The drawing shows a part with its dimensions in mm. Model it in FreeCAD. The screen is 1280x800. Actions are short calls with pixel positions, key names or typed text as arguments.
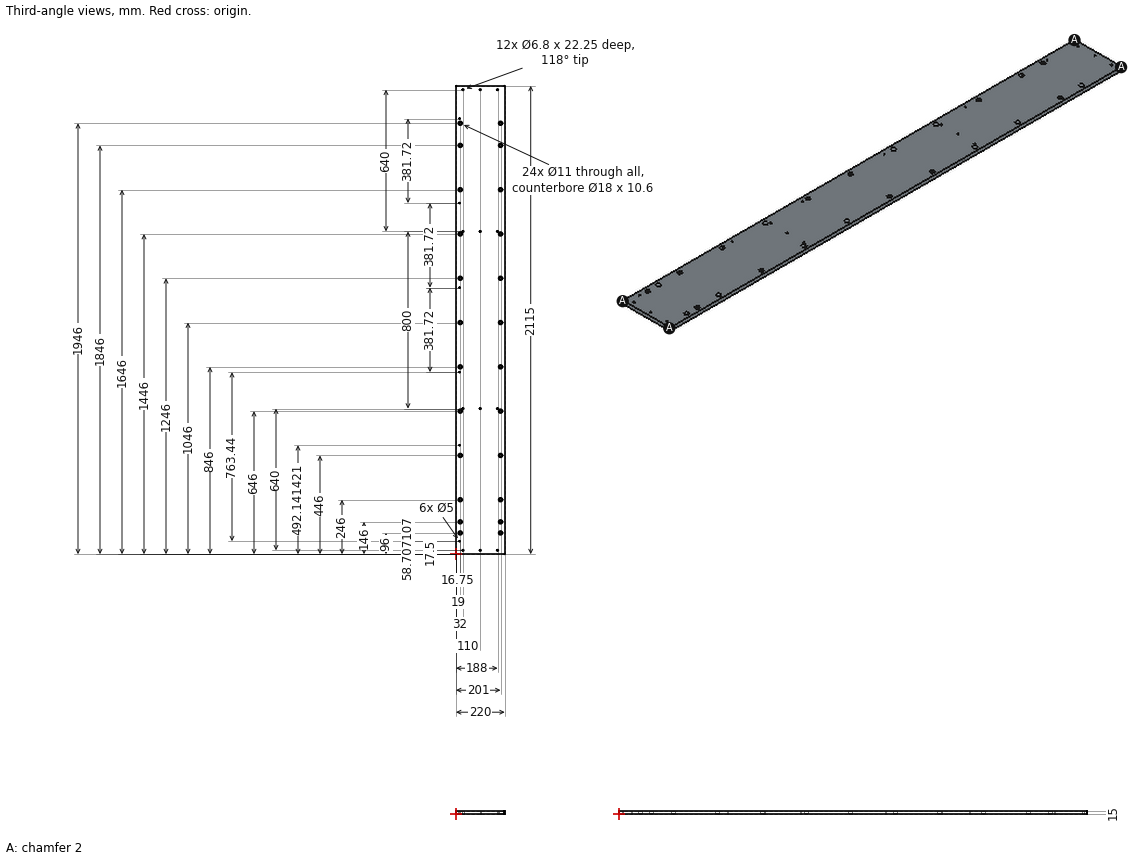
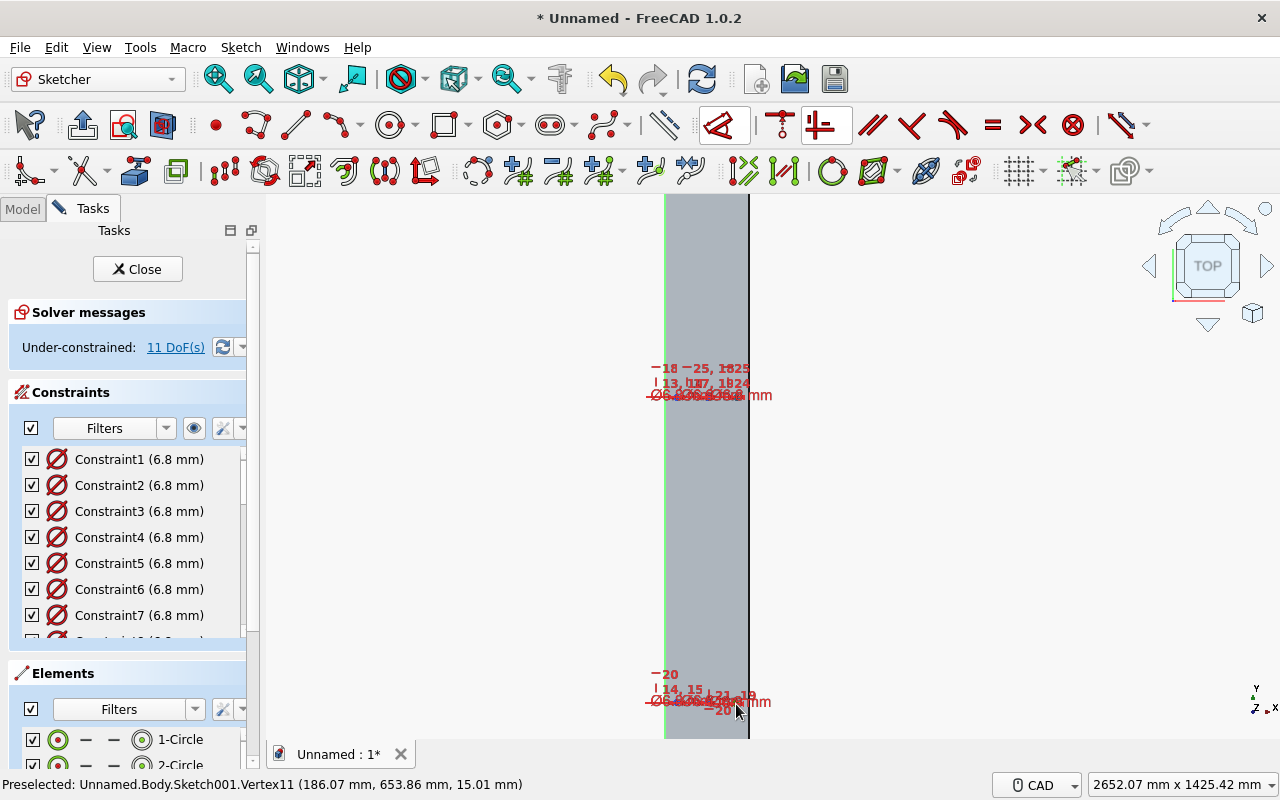
click(846, 126)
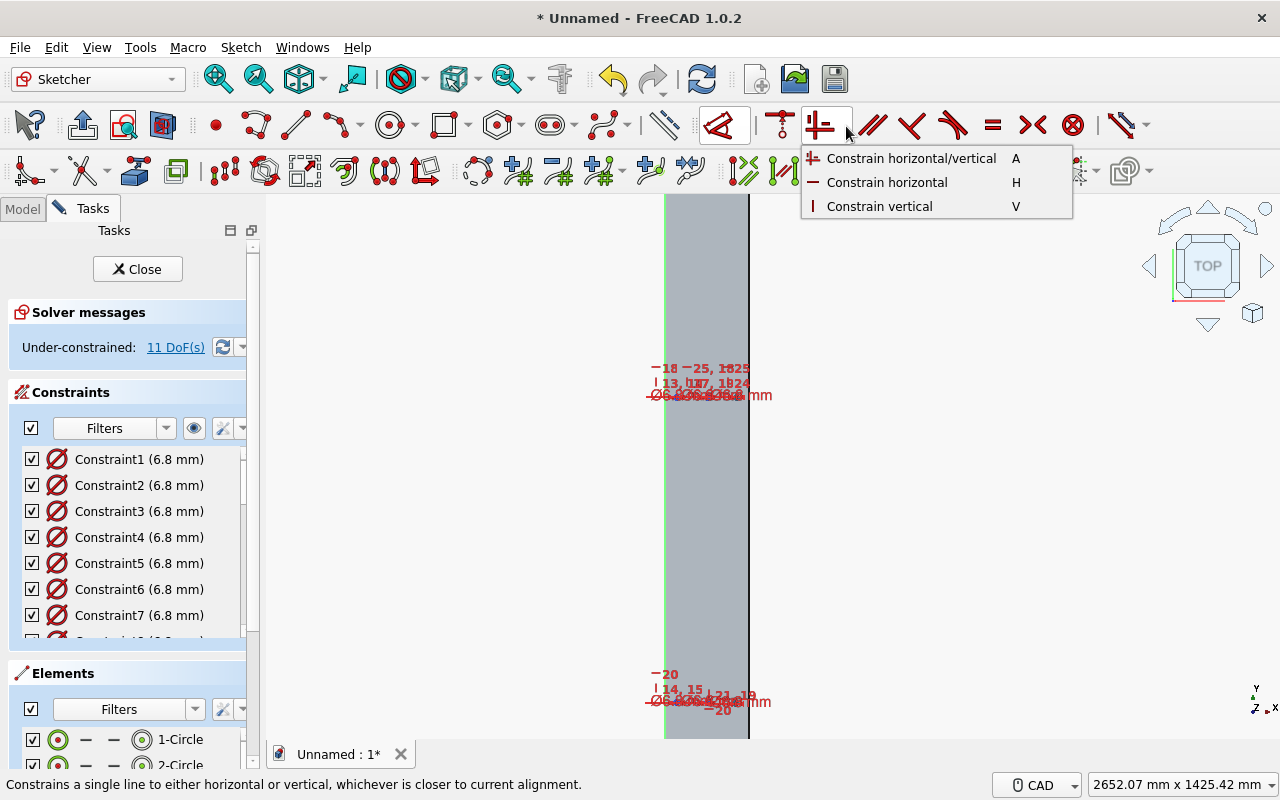
click(937, 206)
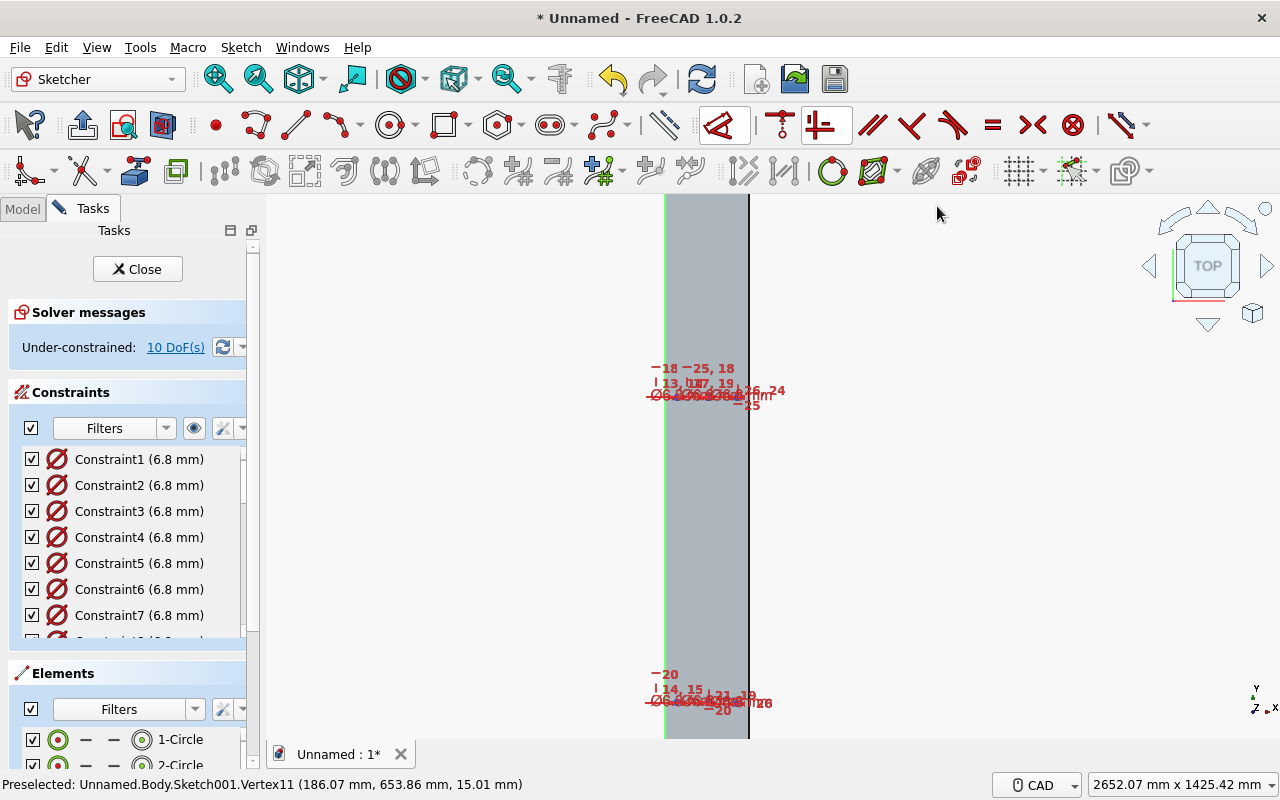
click(707, 703)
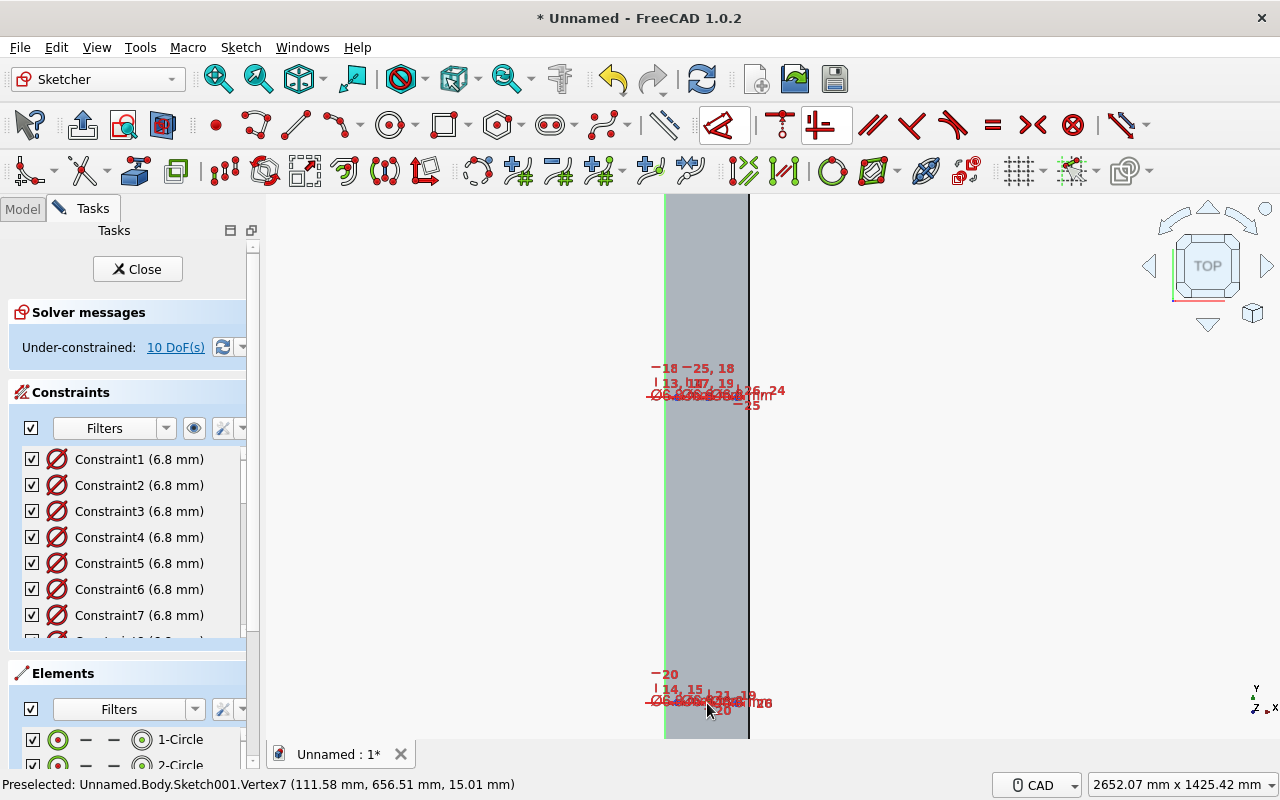
click(737, 704)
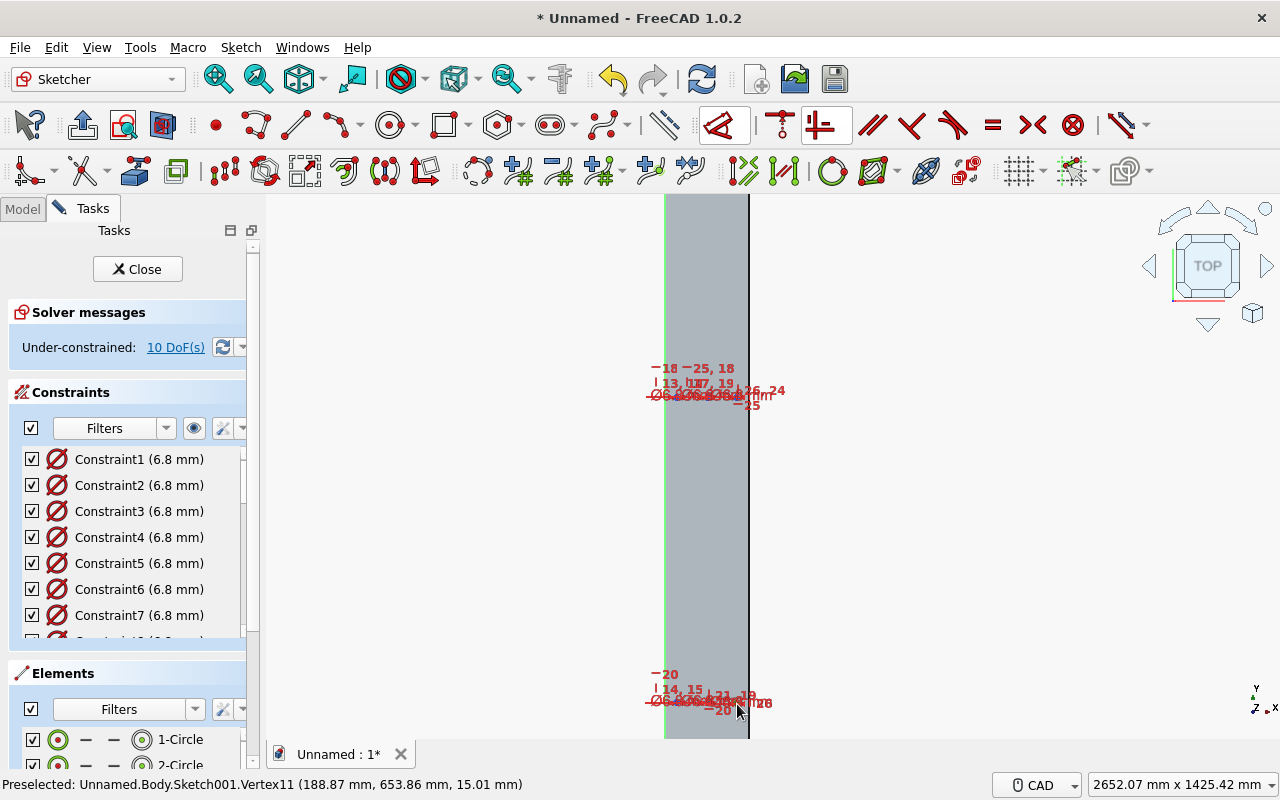
key(h)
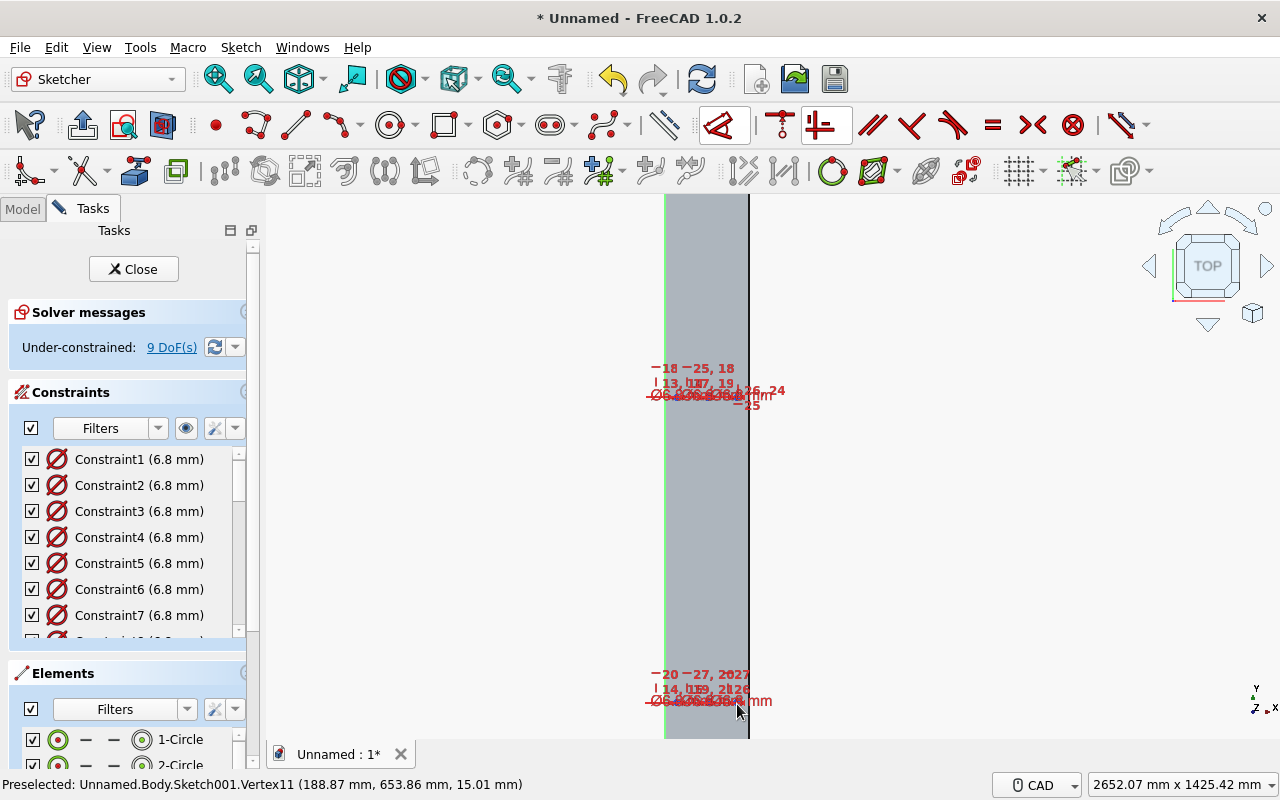
click(737, 703)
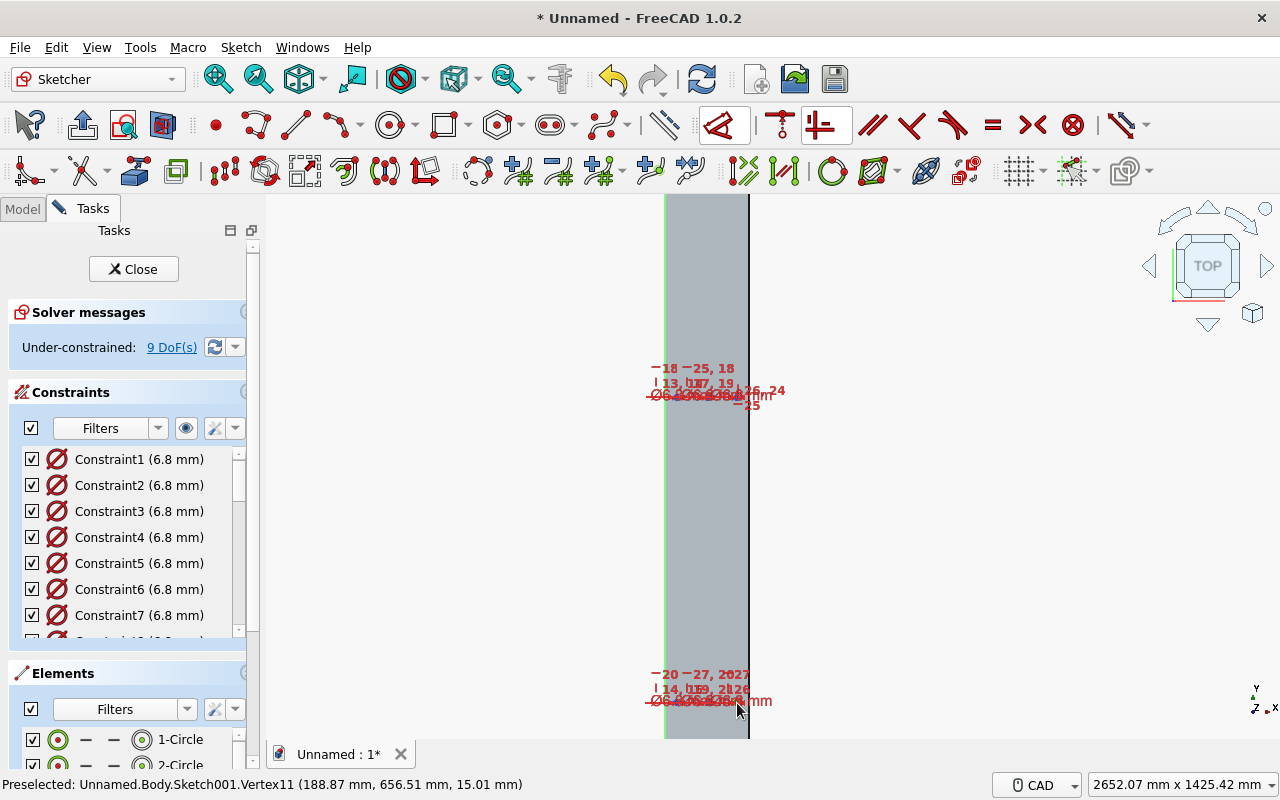
scroll(707, 396, down, 4)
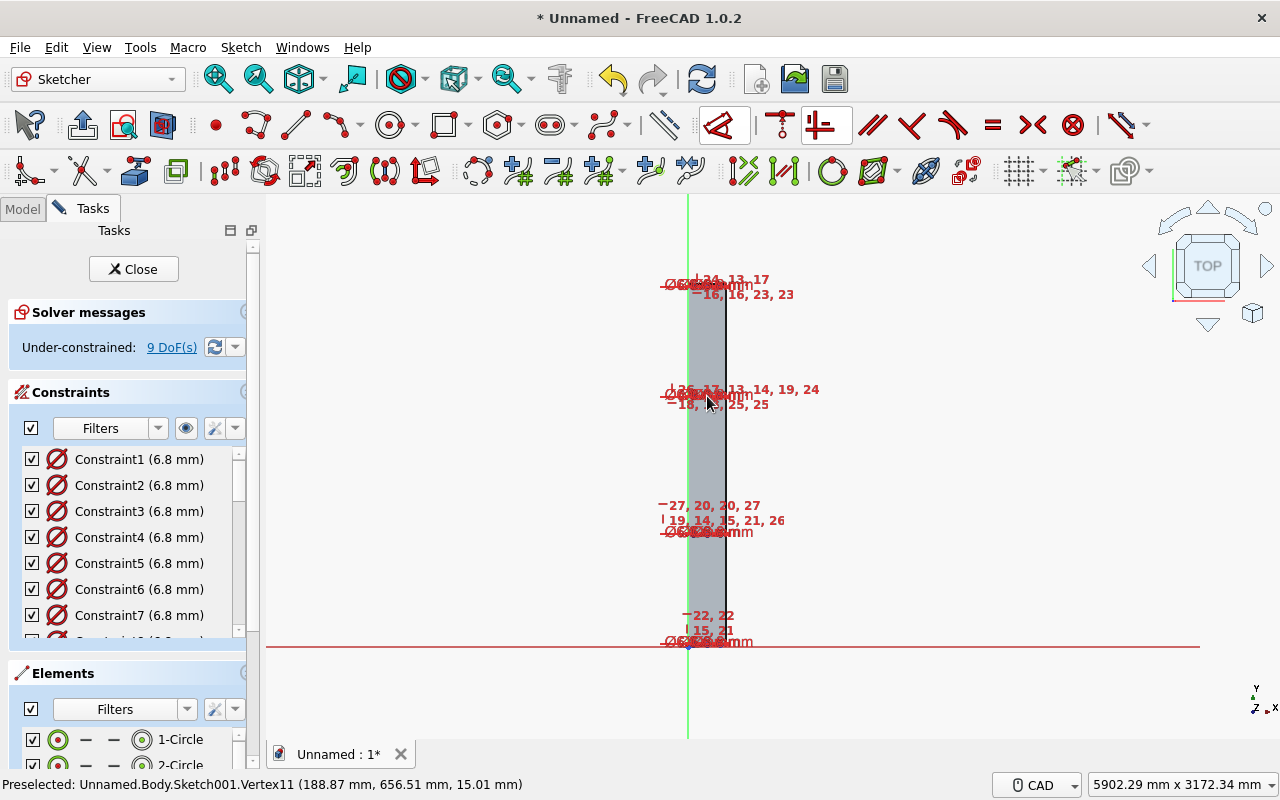
click(721, 644)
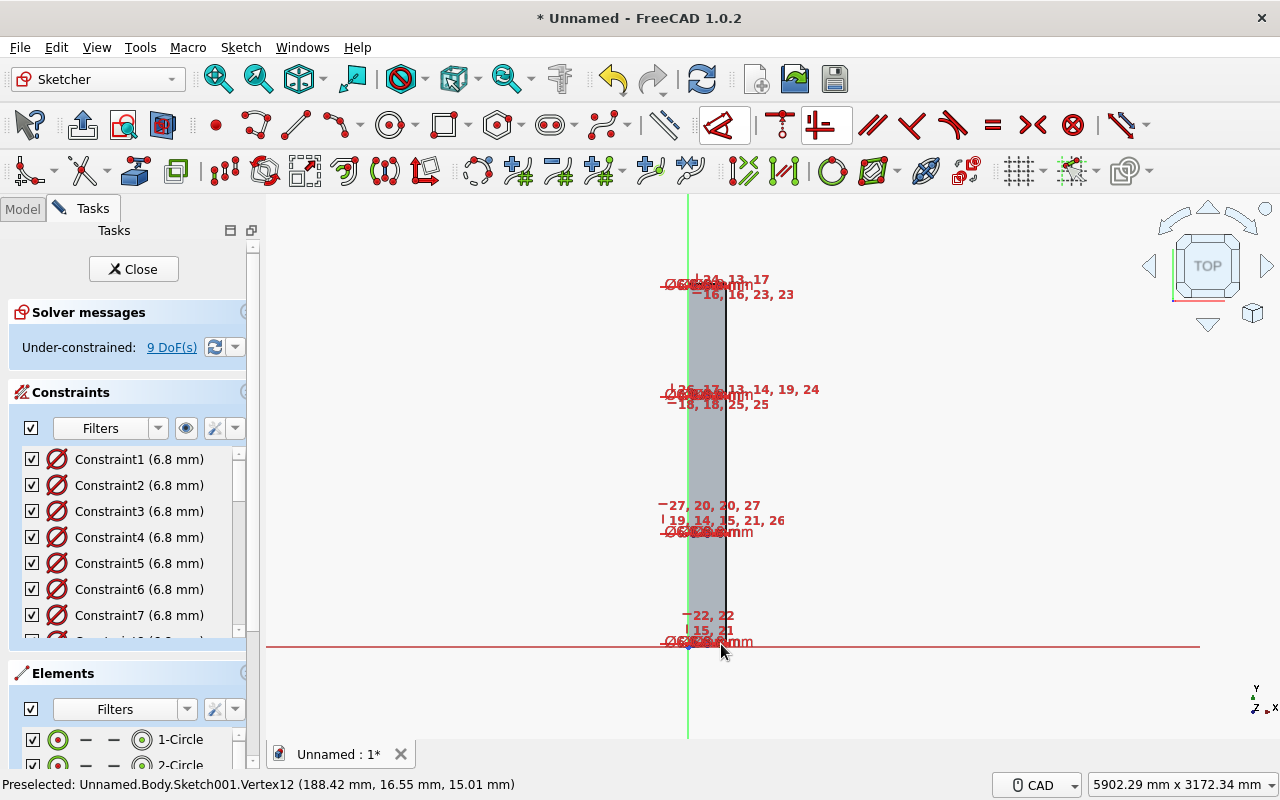
key(v)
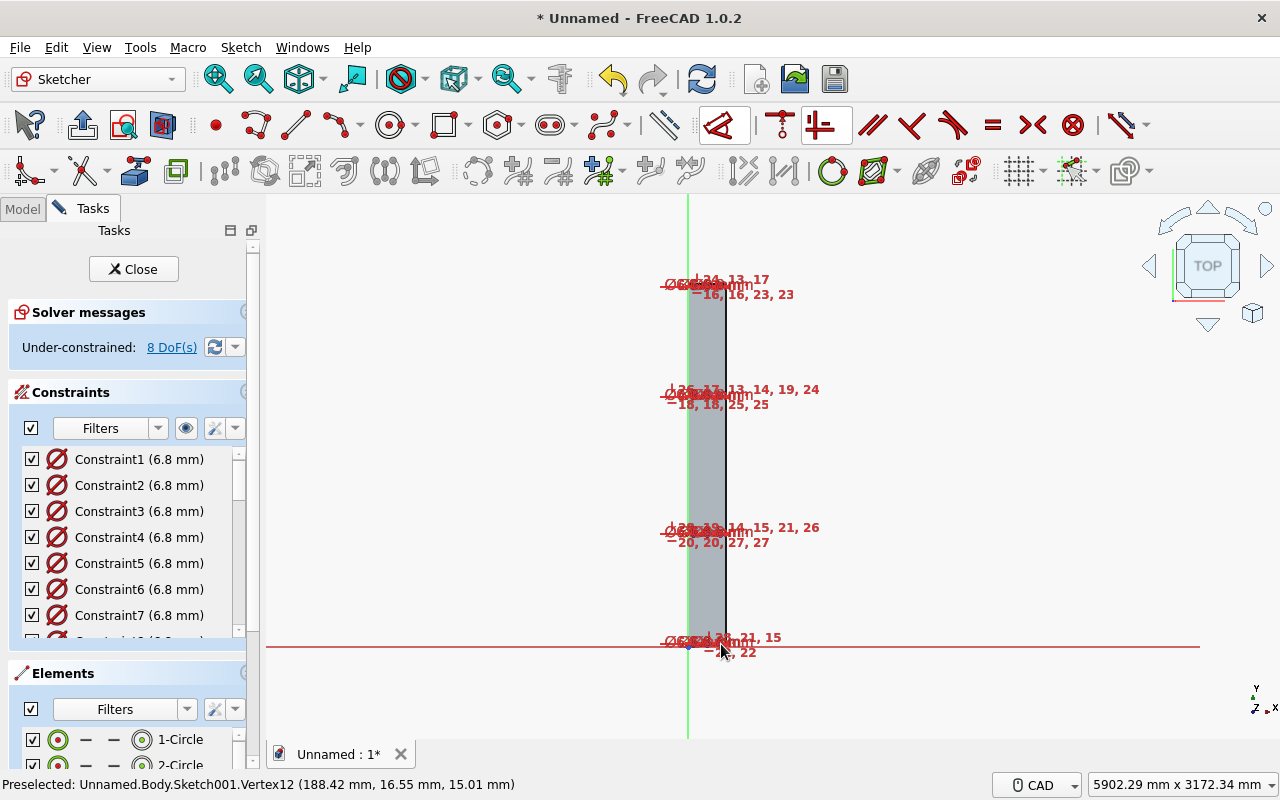
scroll(707, 644, up, 4)